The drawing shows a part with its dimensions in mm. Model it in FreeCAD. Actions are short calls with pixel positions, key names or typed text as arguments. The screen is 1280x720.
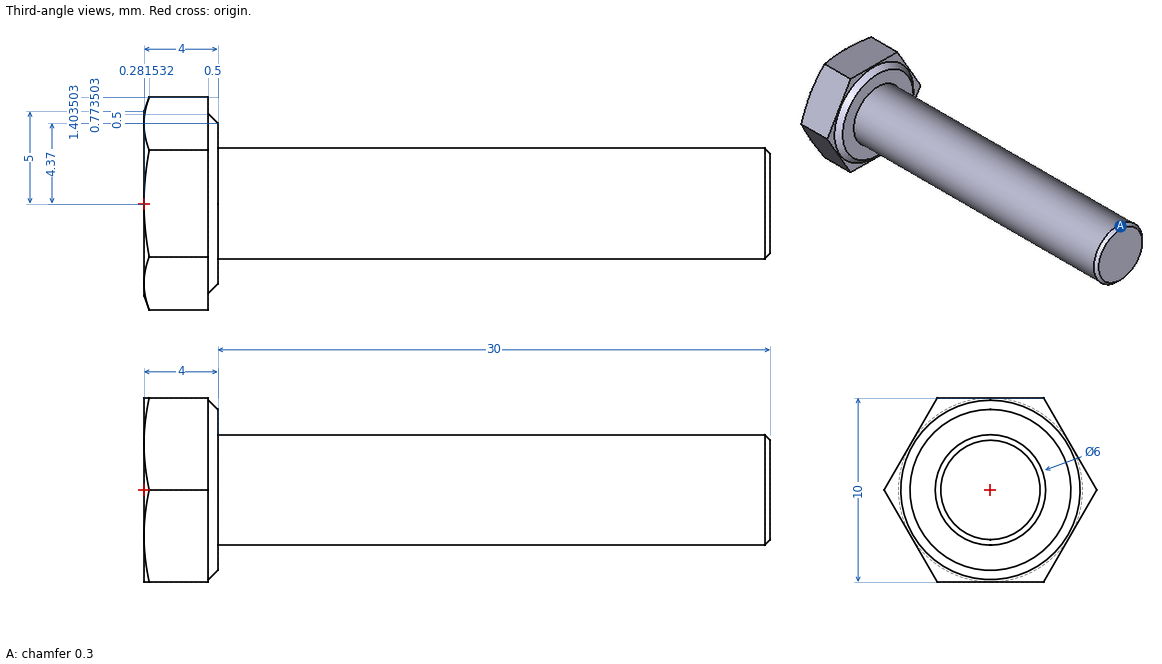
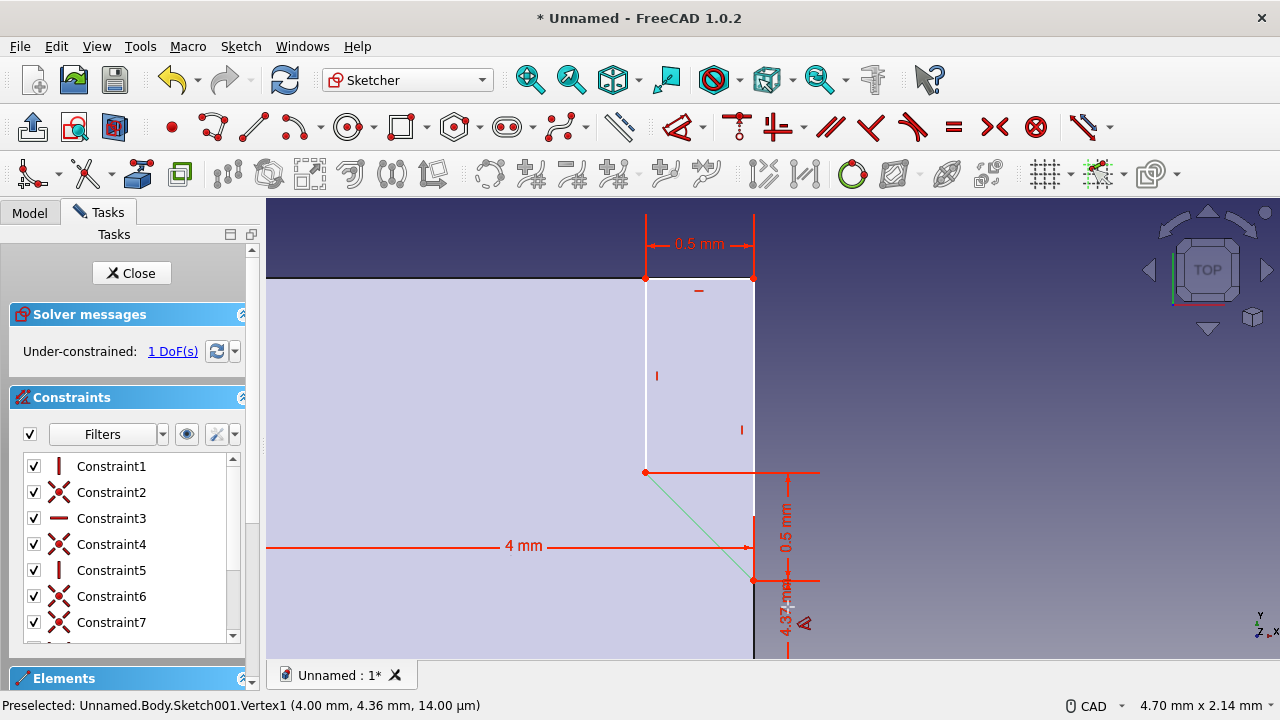
click(754, 490)
click(788, 430)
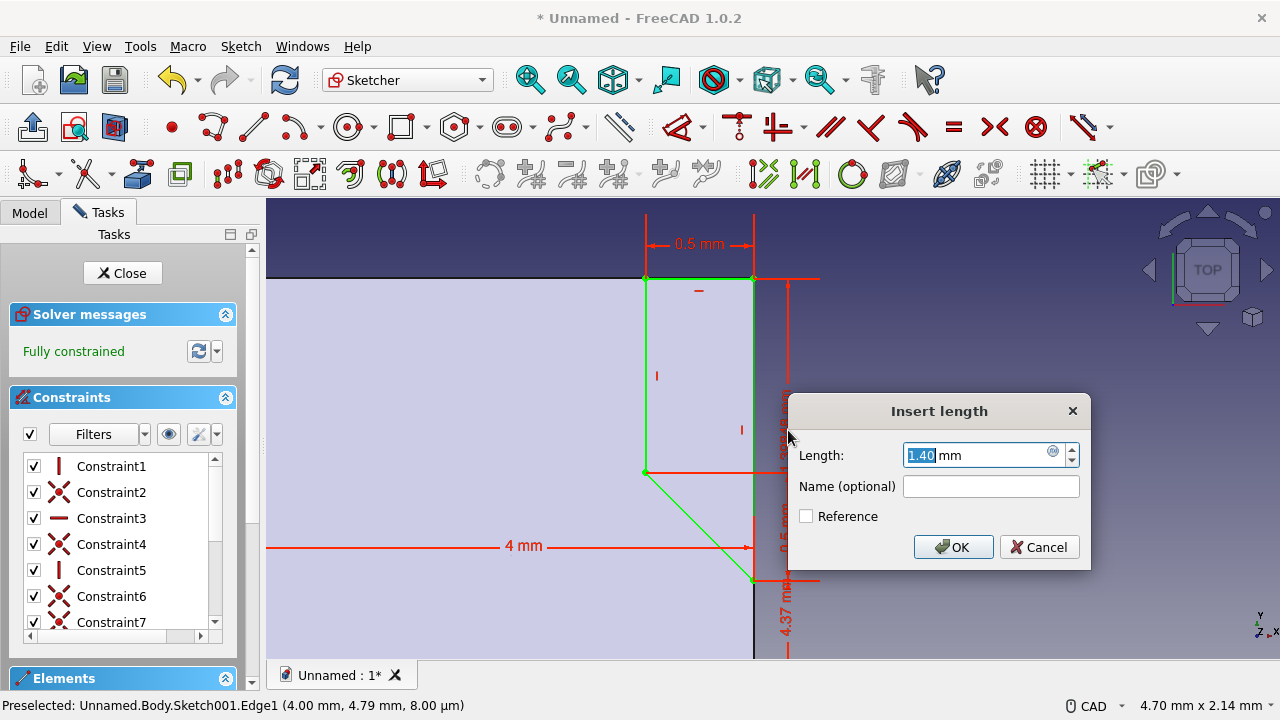
text(1.403503)
key(Return)
key(Escape)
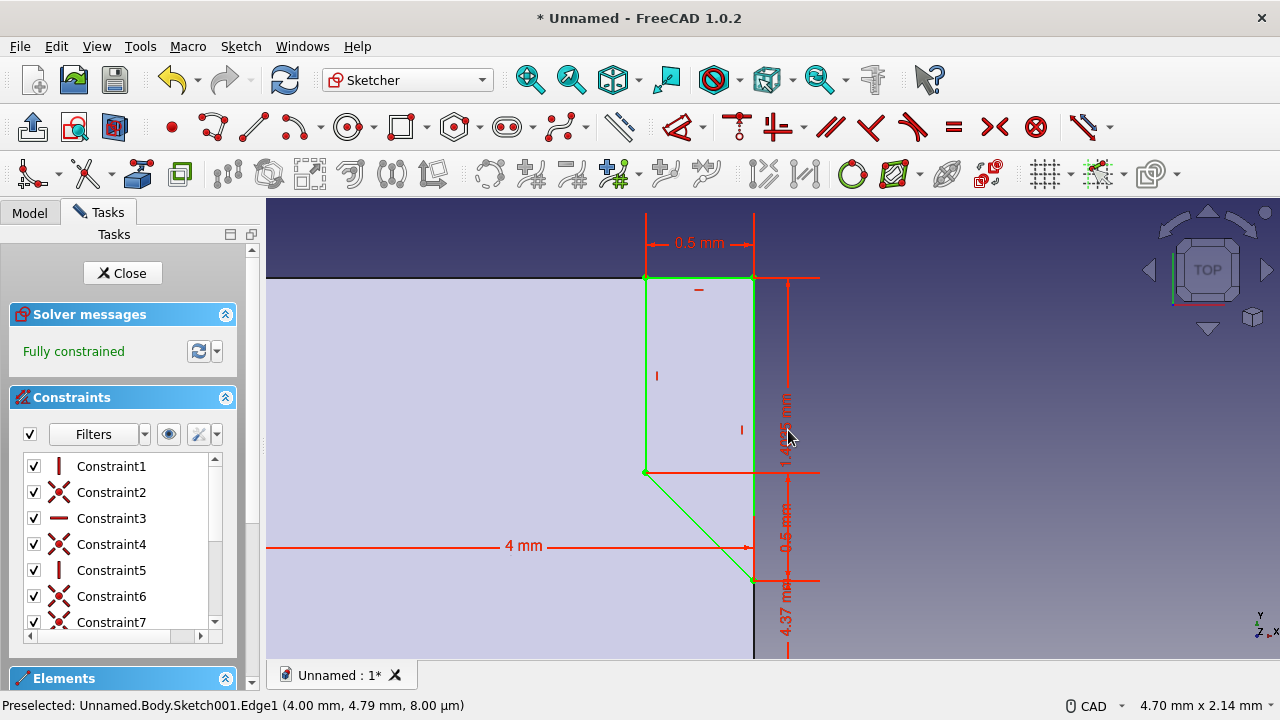
click(123, 273)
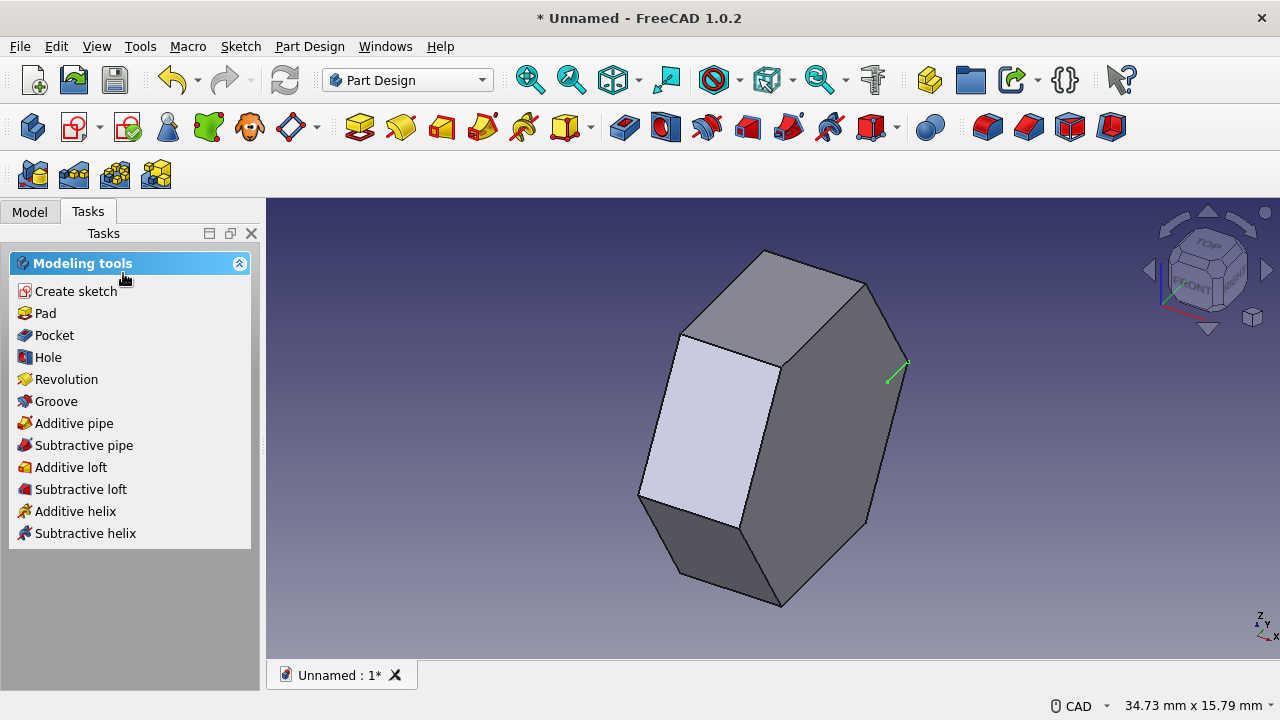
click(707, 128)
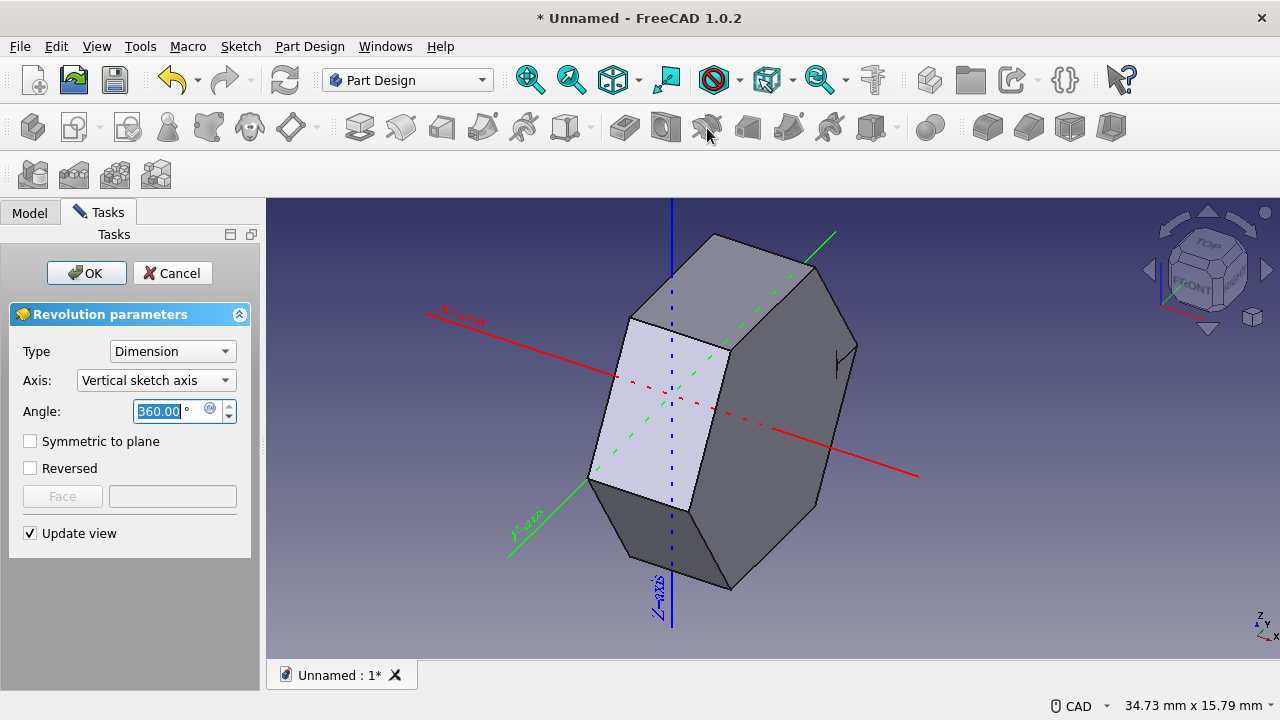
click(157, 380)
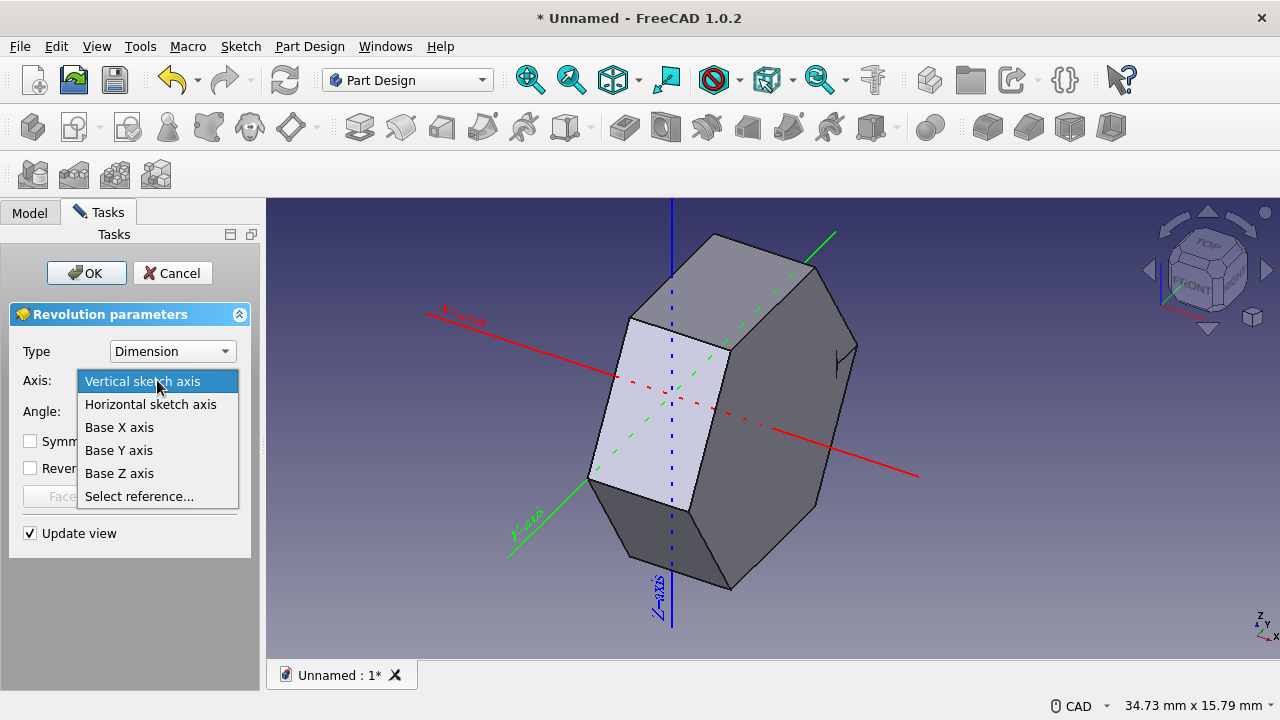
click(156, 404)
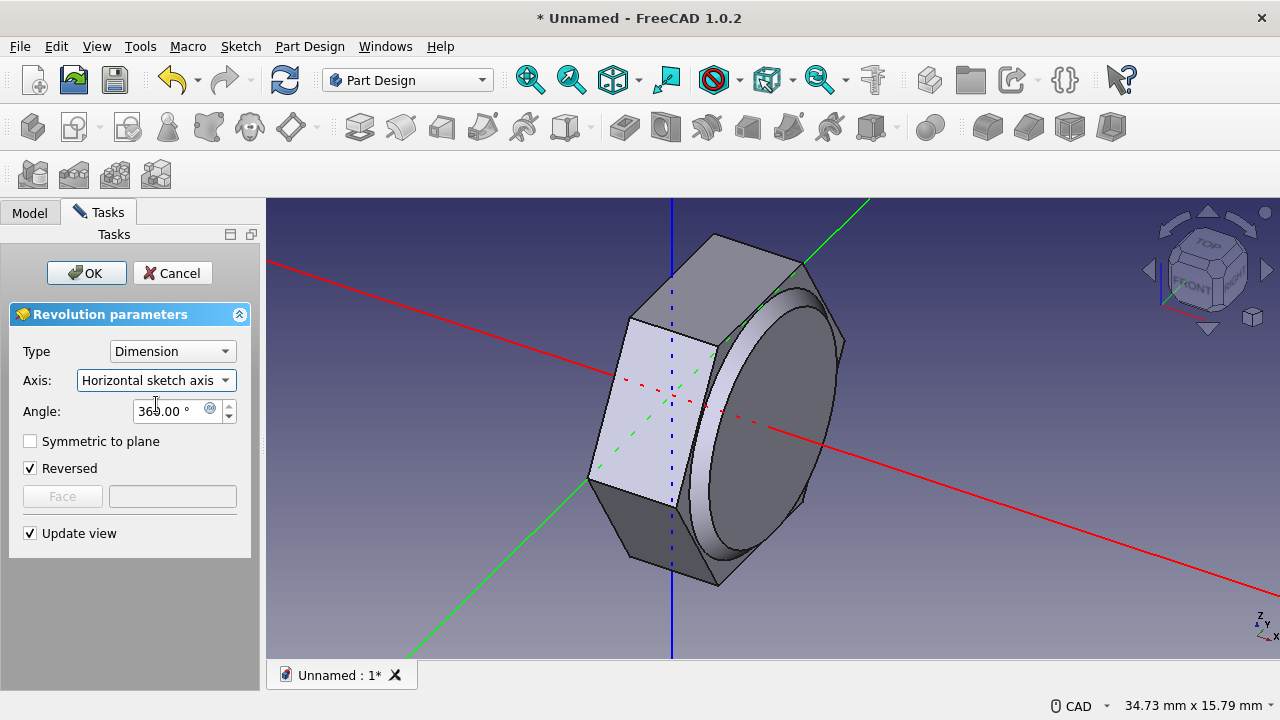
click(87, 273)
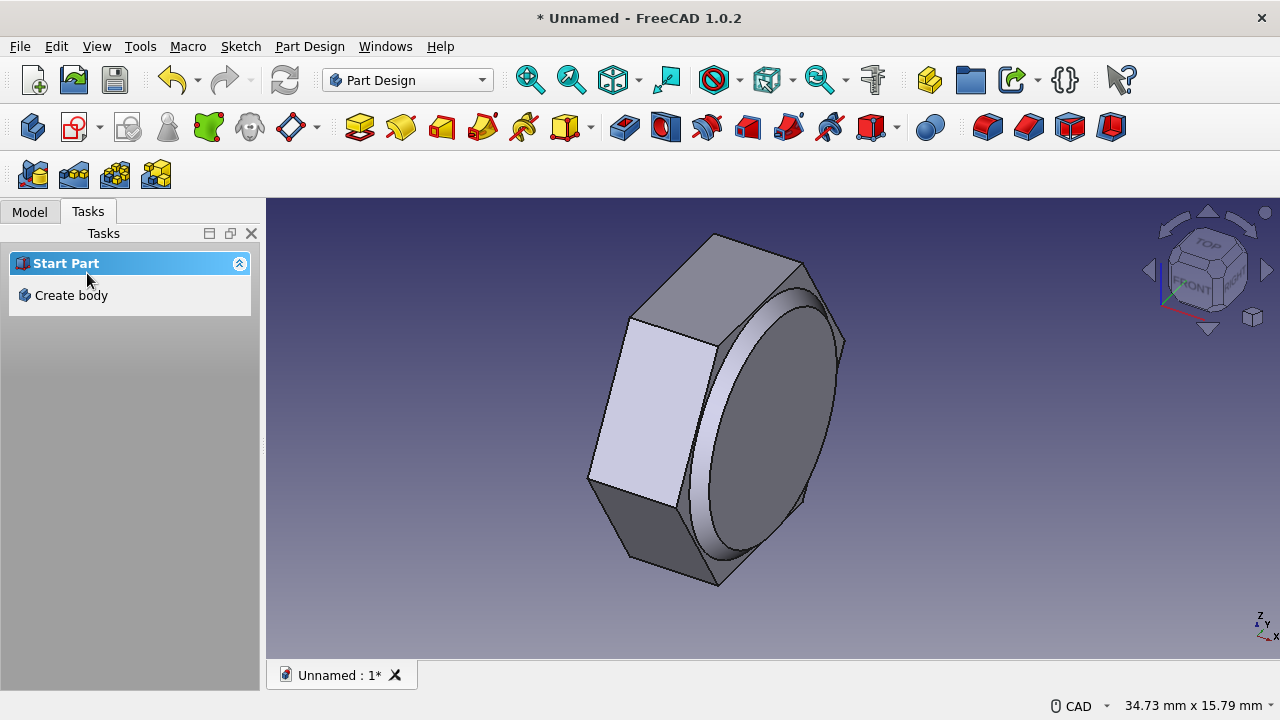
click(531, 80)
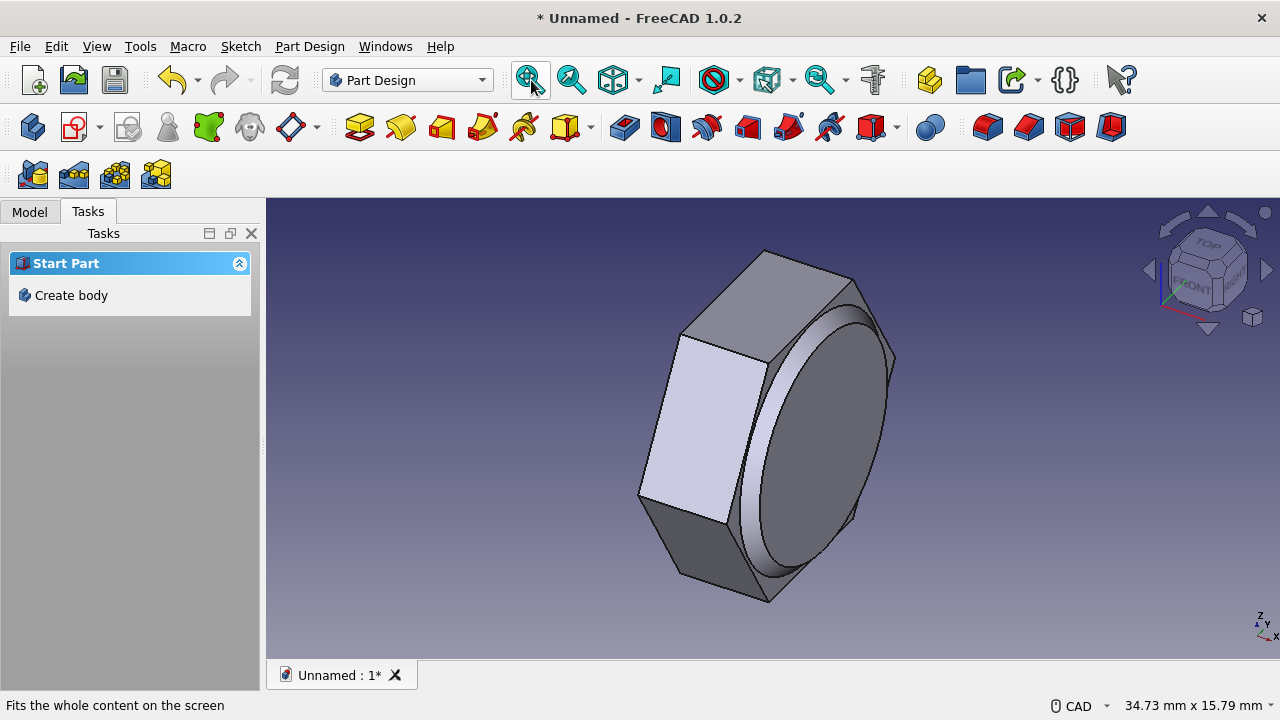
click(74, 128)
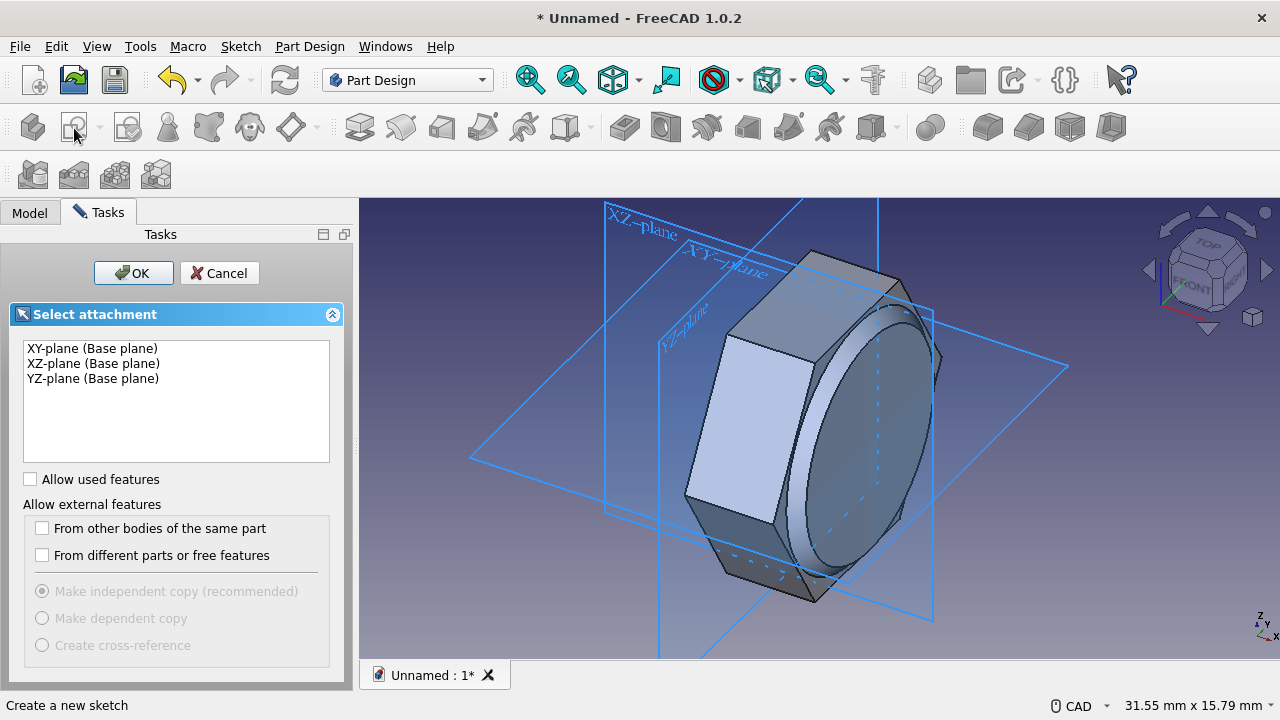
click(84, 348)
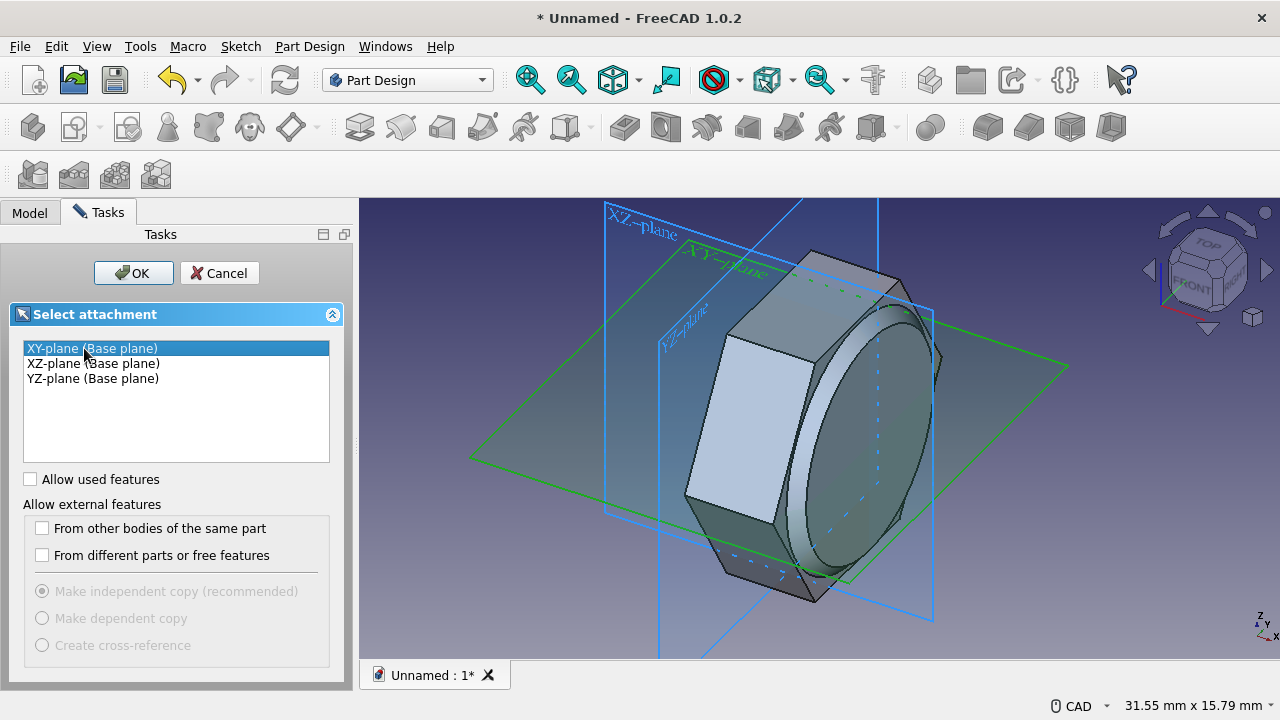
click(134, 273)